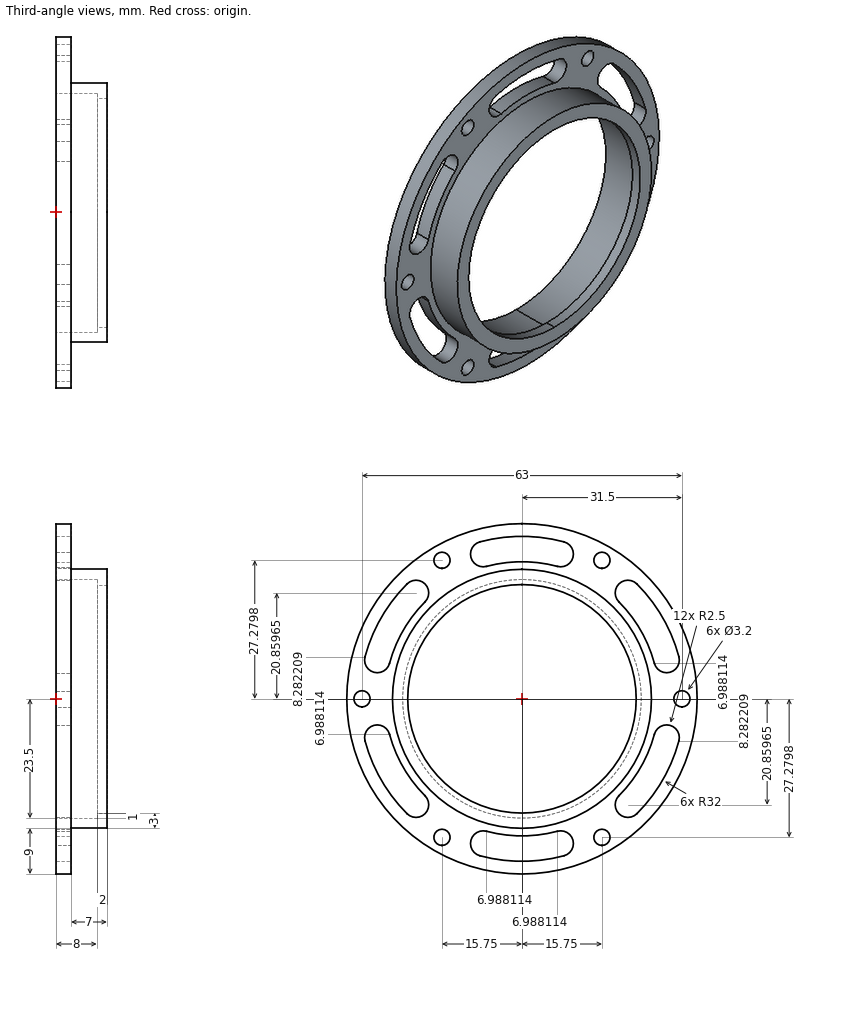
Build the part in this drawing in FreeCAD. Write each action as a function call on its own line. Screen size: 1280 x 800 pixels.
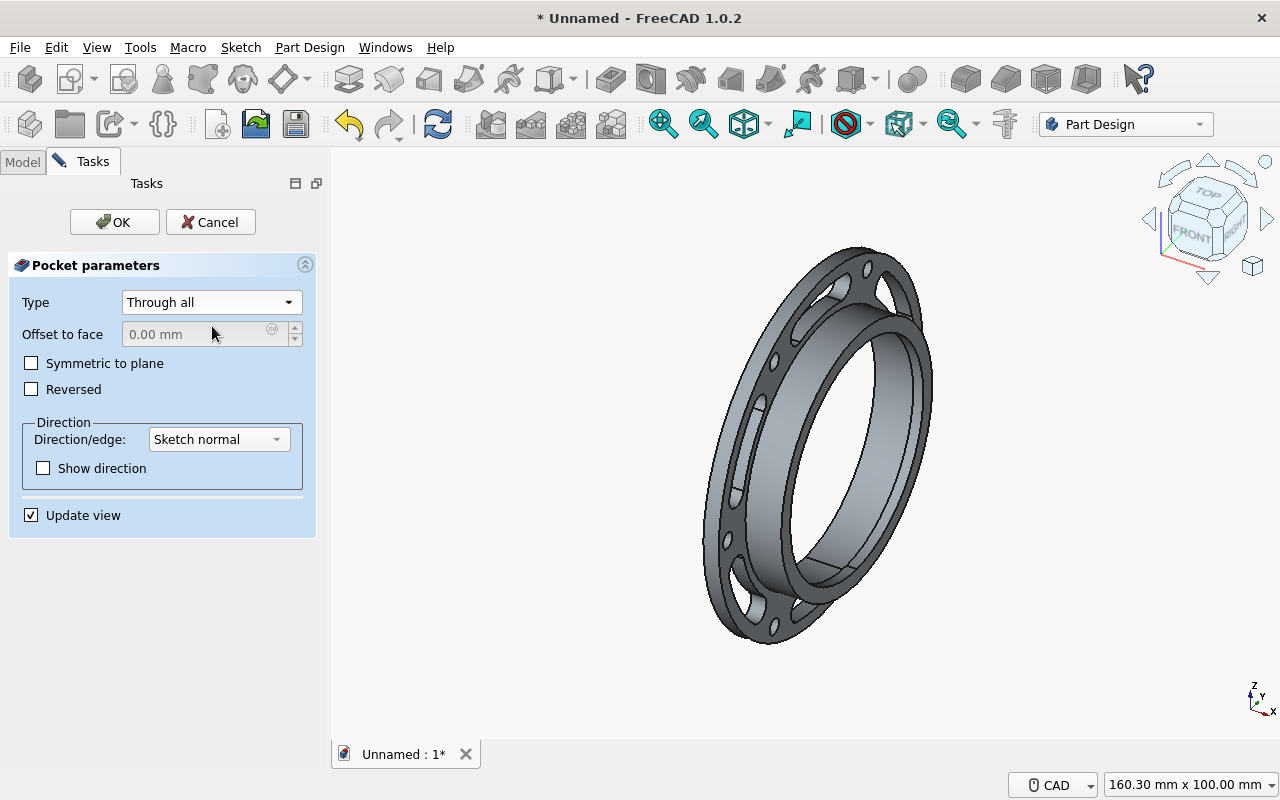
click(115, 222)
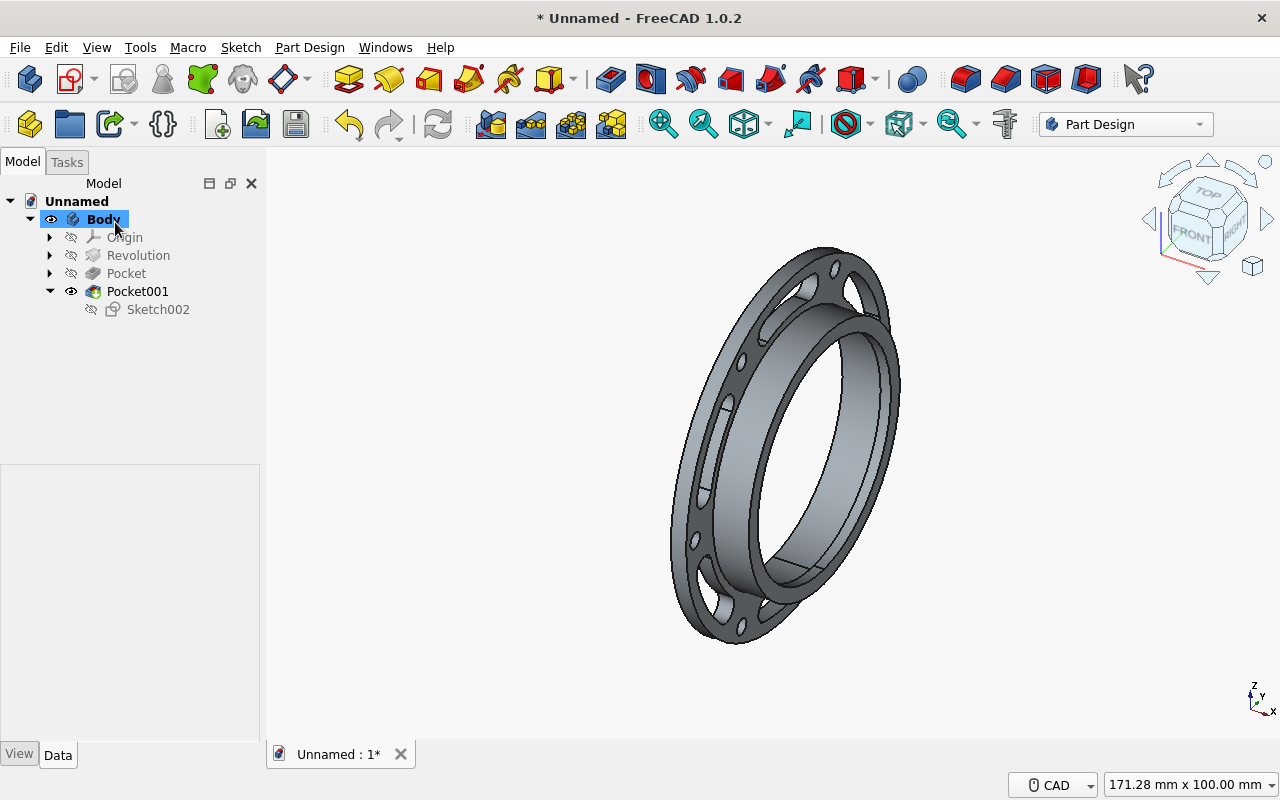
key(0)